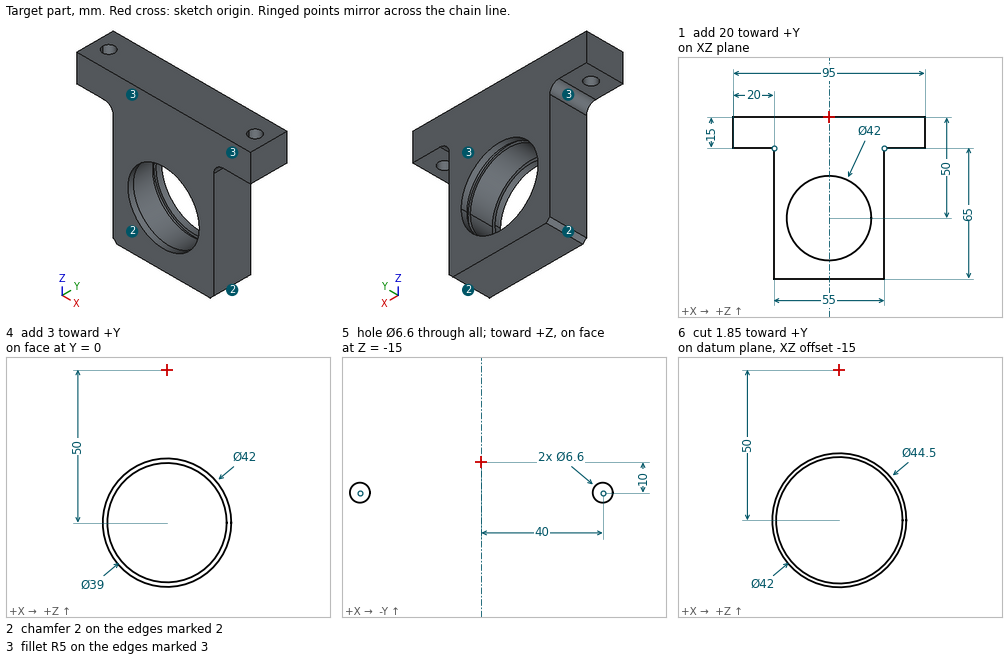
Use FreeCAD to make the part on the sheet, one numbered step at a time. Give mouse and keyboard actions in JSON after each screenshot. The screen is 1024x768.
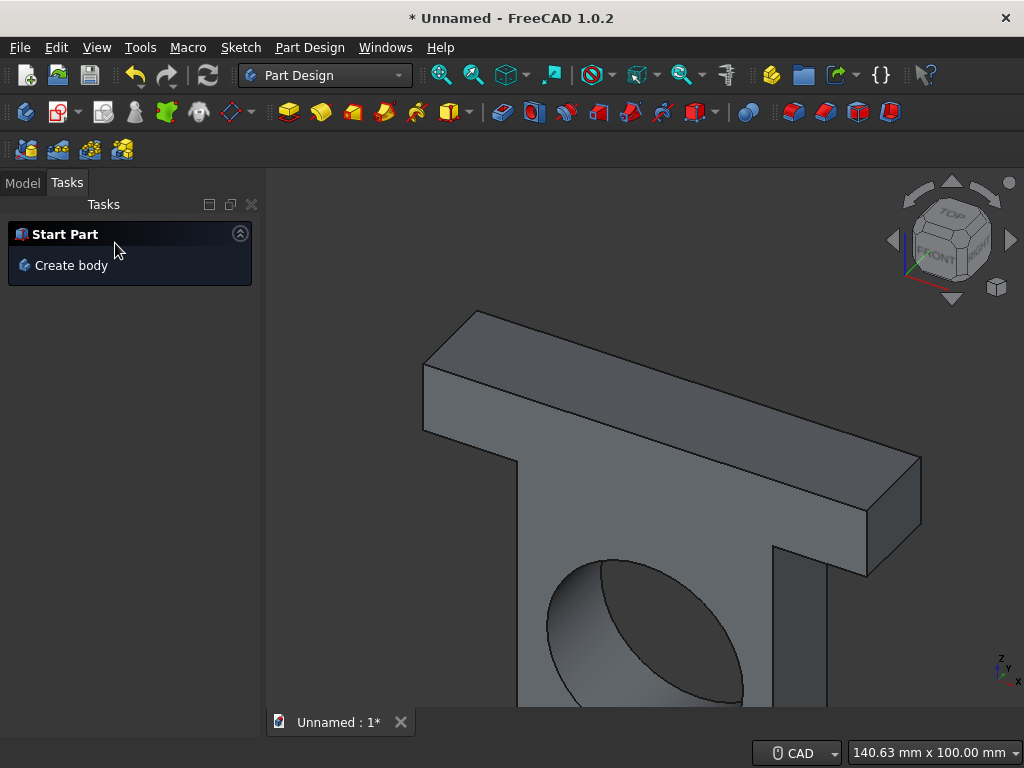
{"action": "left_click", "coordinate": [442, 76]}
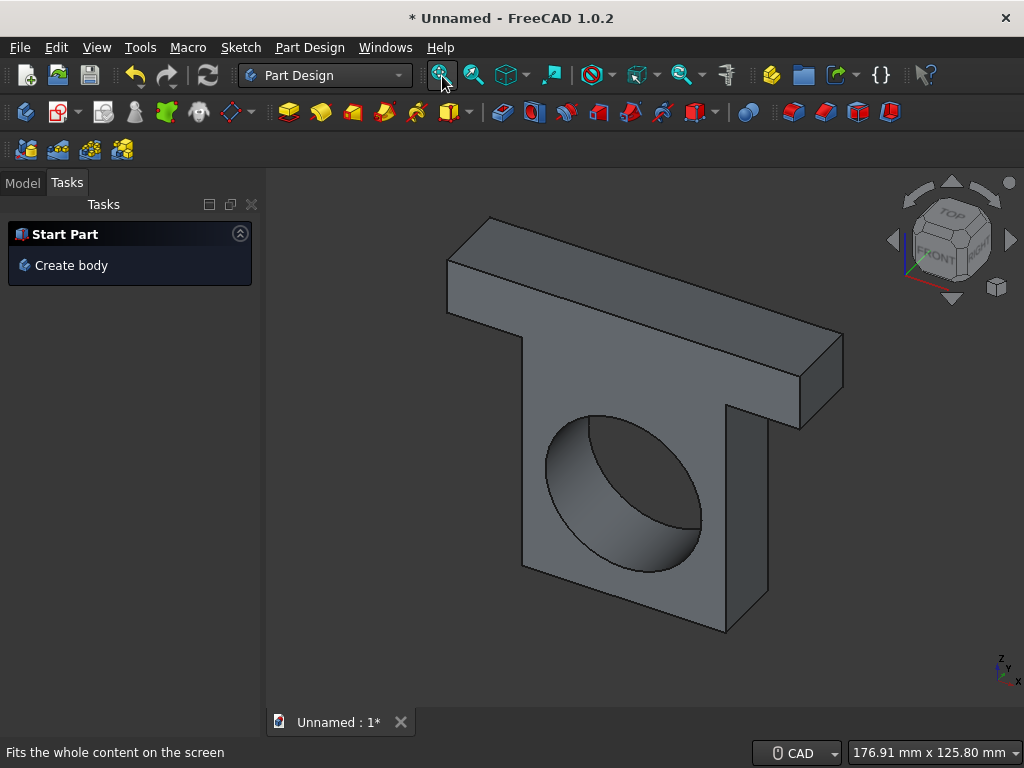
{"action": "key", "text": "0"}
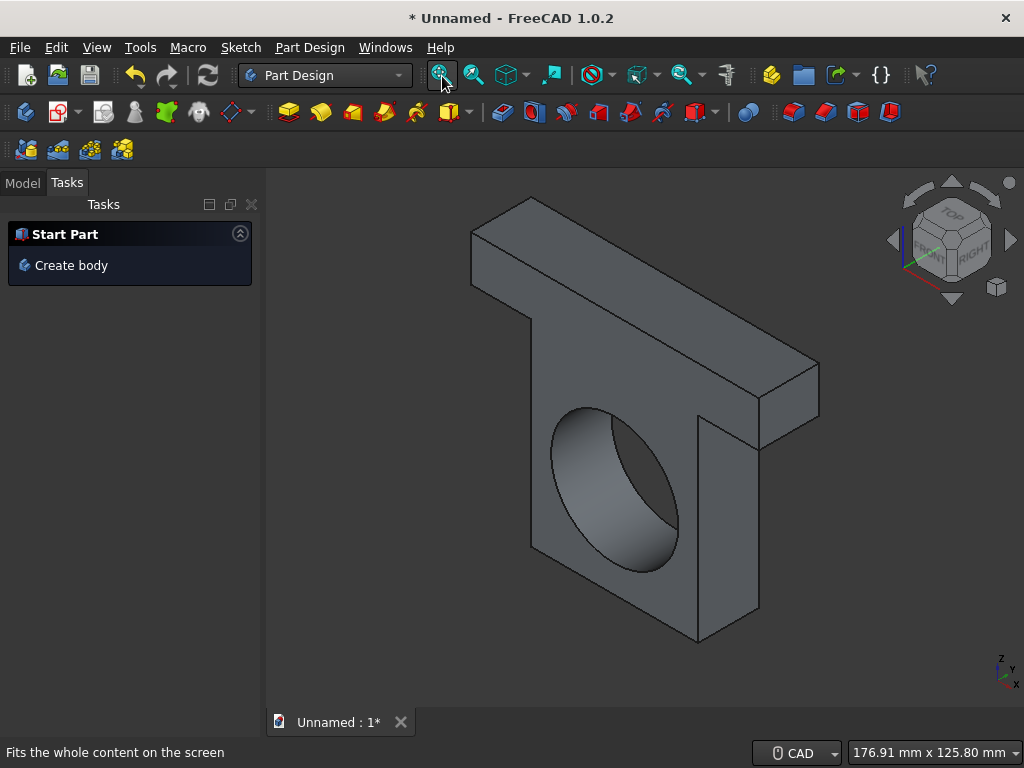
{"action": "key", "text": "2"}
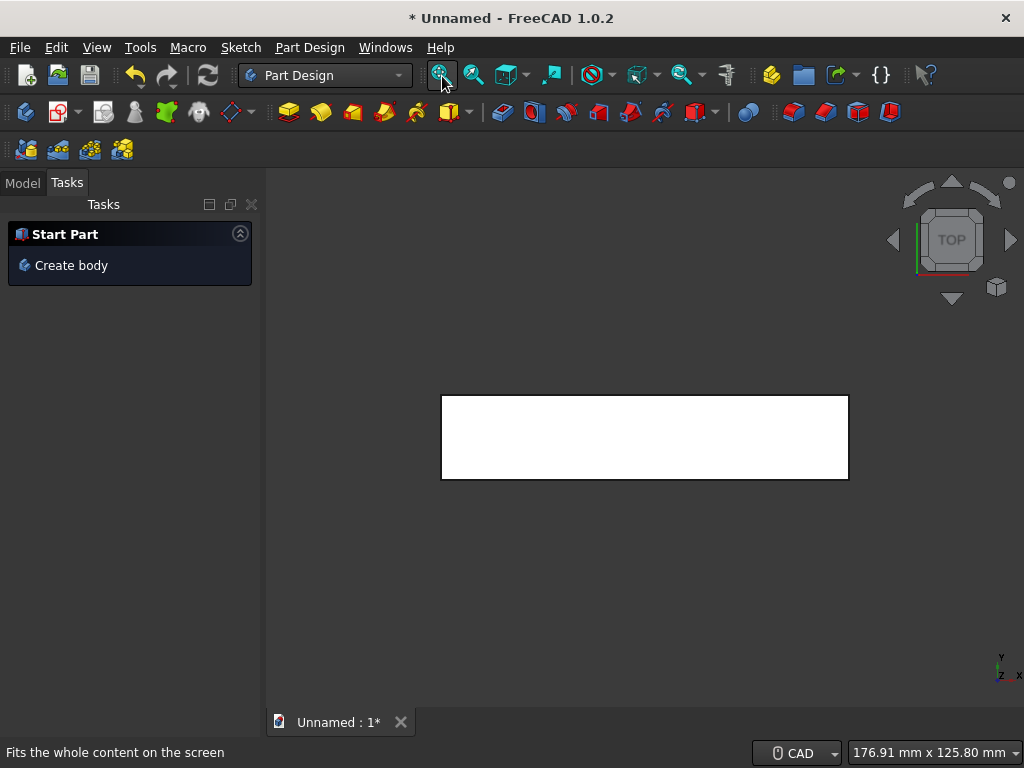
{"action": "key", "text": "1"}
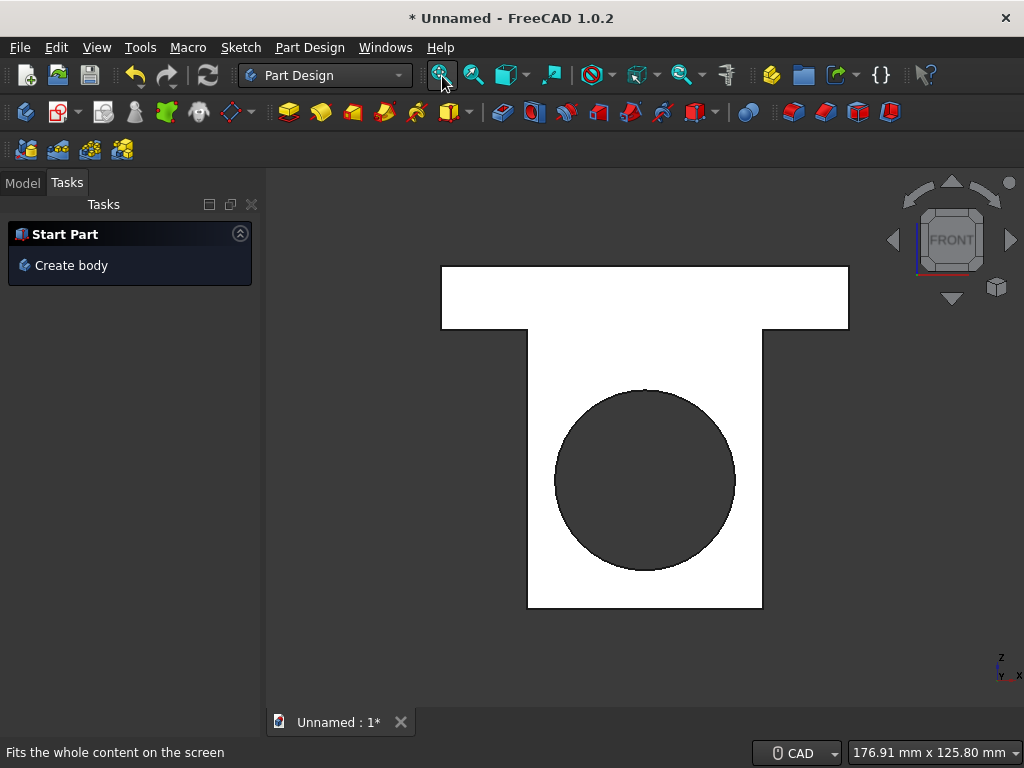
{"action": "key", "text": "3"}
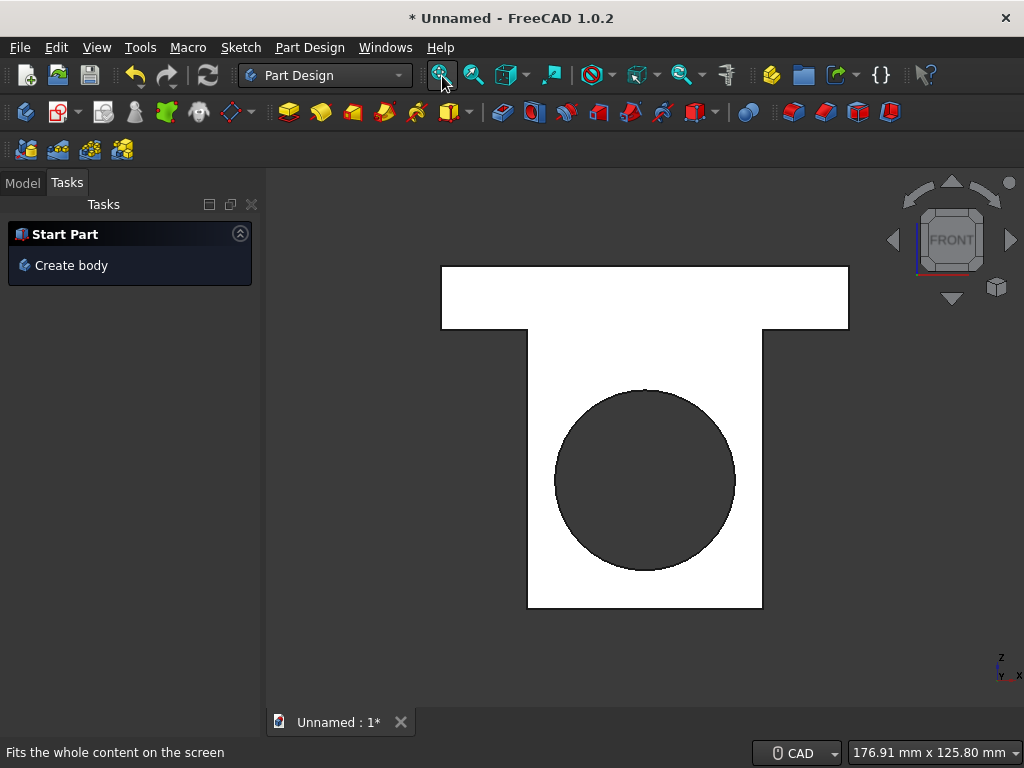
{"action": "left_click", "coordinate": [645, 608]}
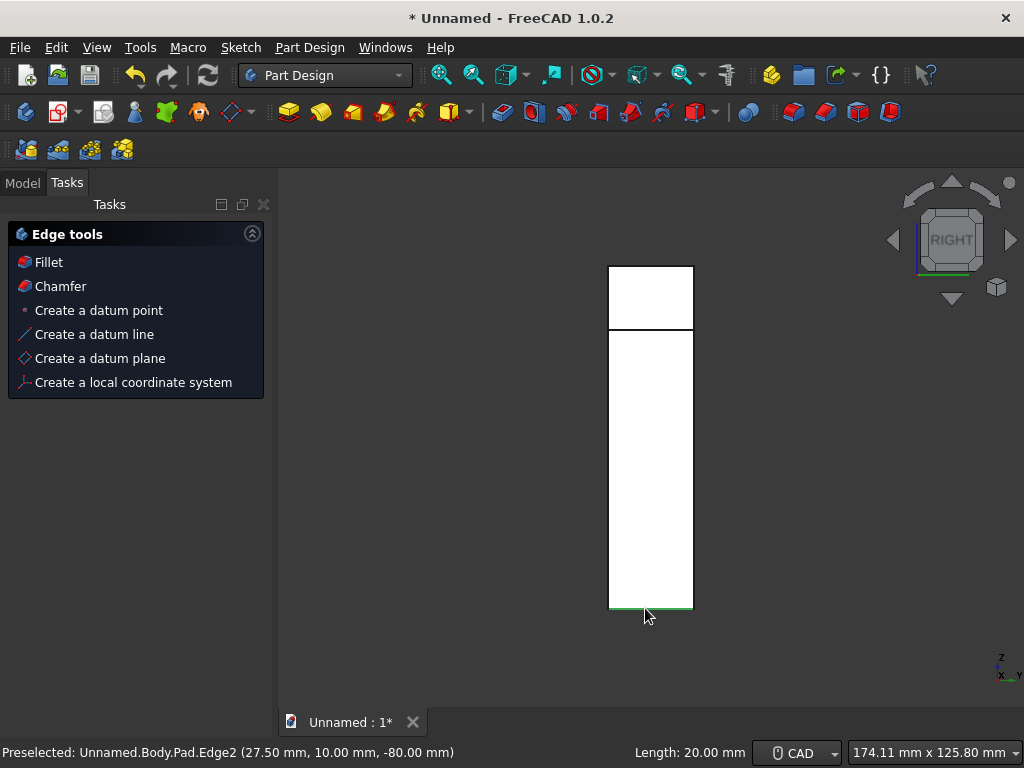
{"action": "key", "text": "5"}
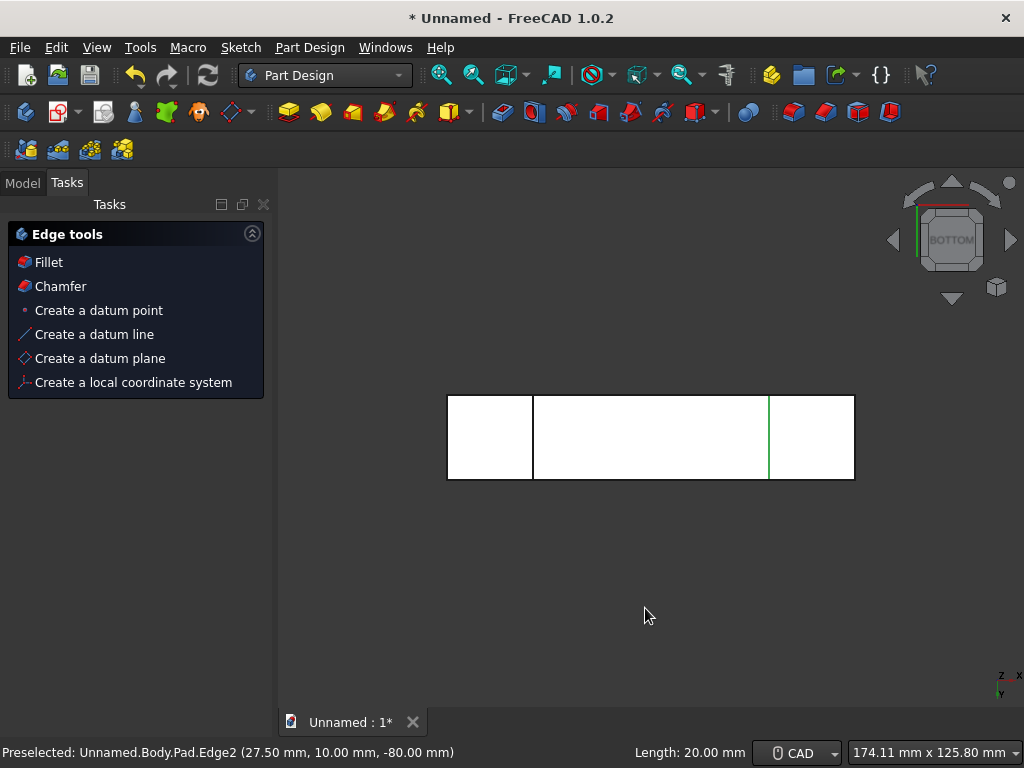
{"action": "left_click", "coordinate": [533, 436], "text": "ctrl"}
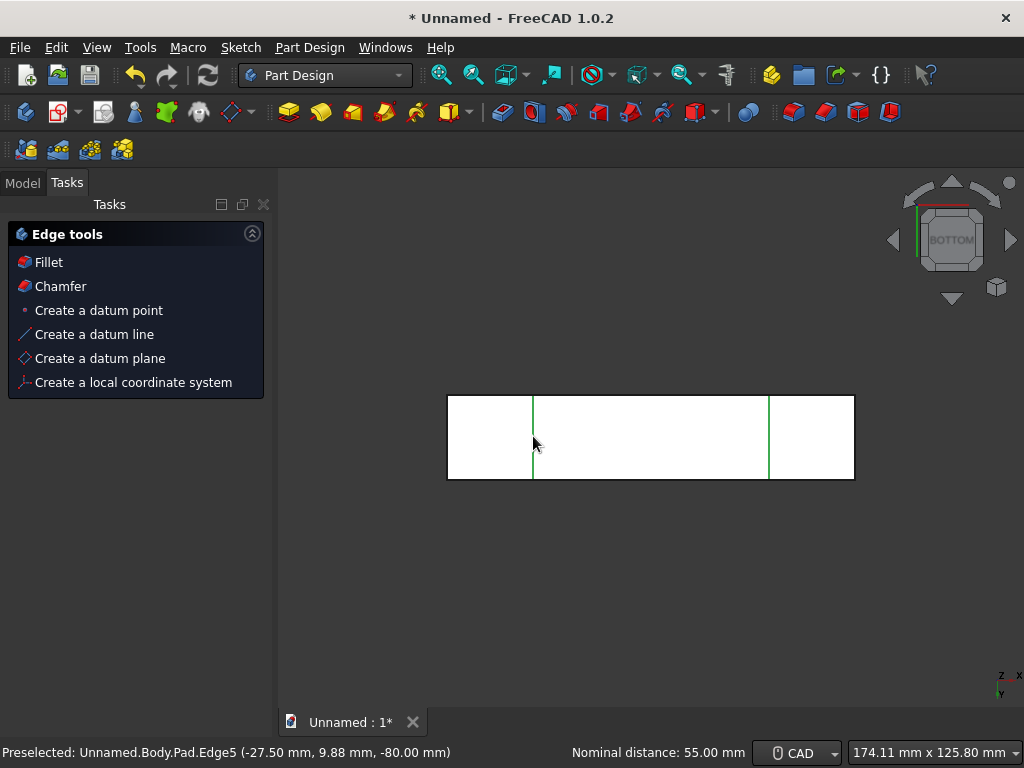
{"action": "left_click", "coordinate": [826, 112]}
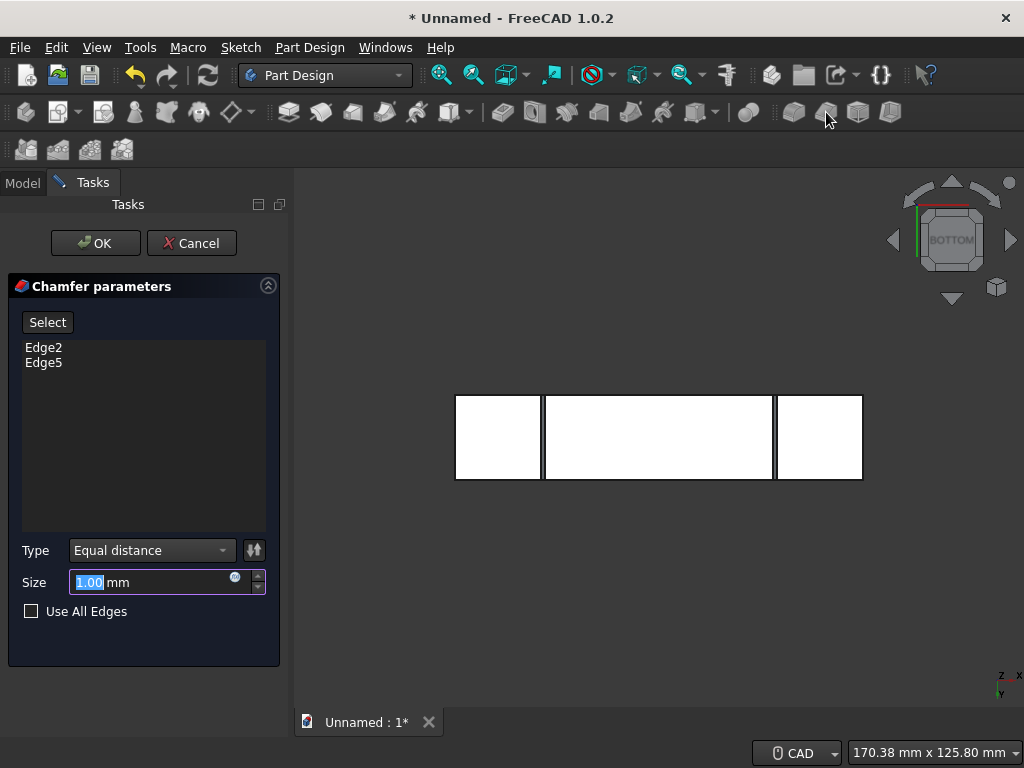
{"action": "type", "text": "2"}
{"action": "key", "text": "Tab"}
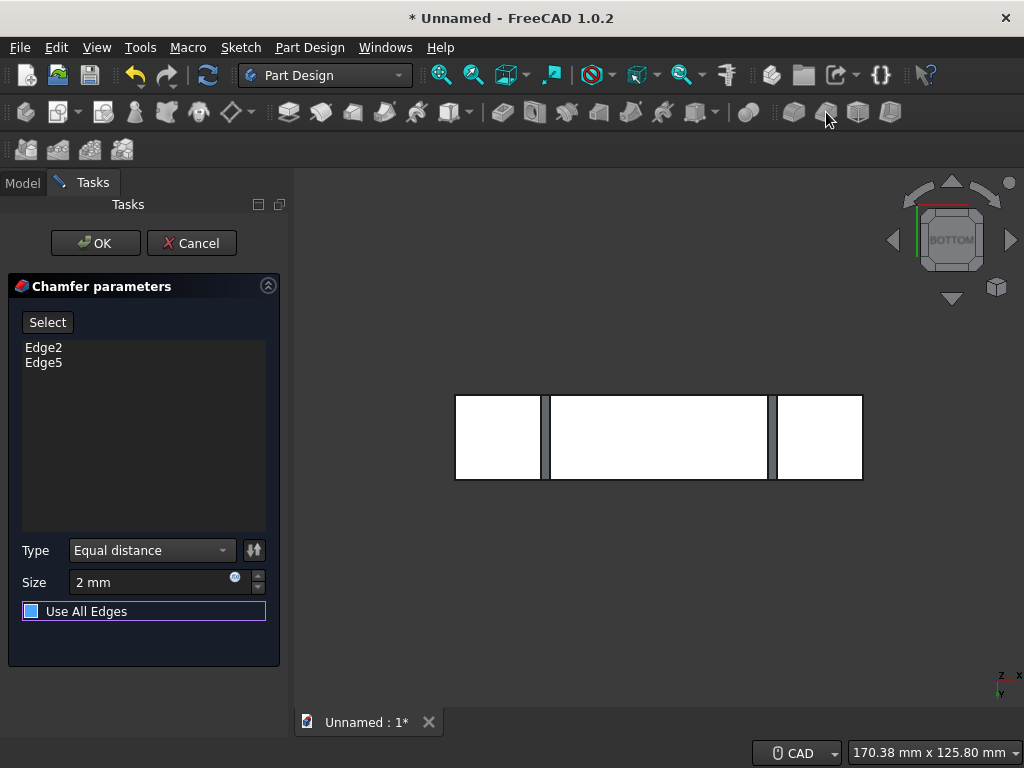
{"action": "left_click", "coordinate": [96, 243]}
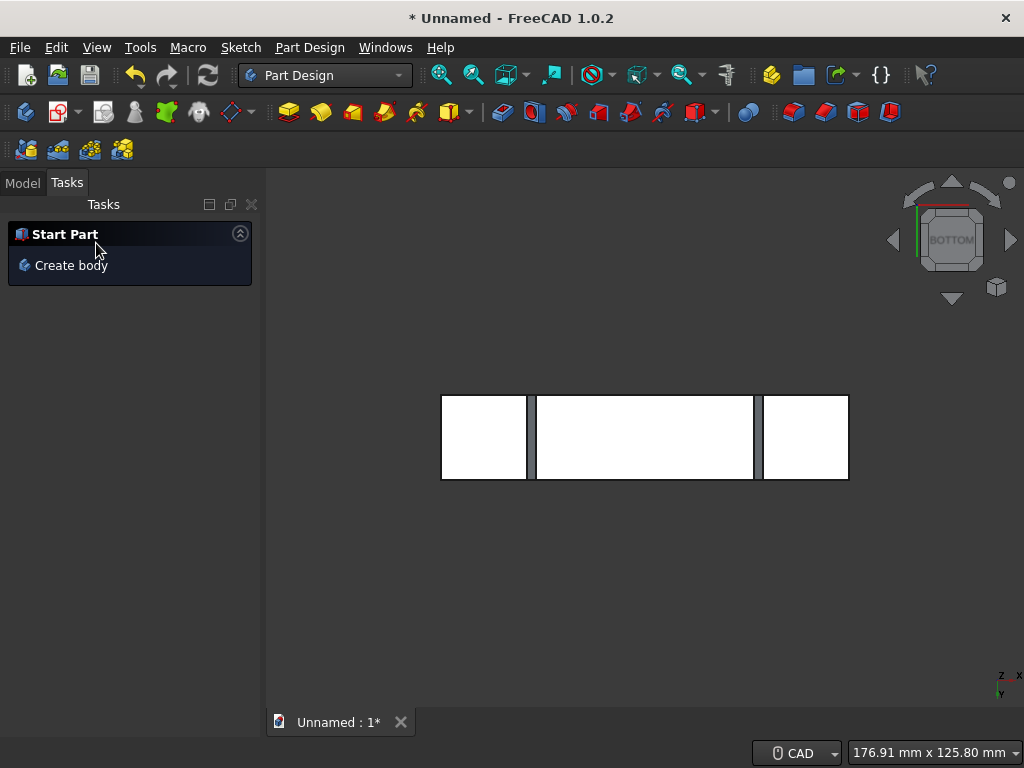
{"action": "key", "text": "0"}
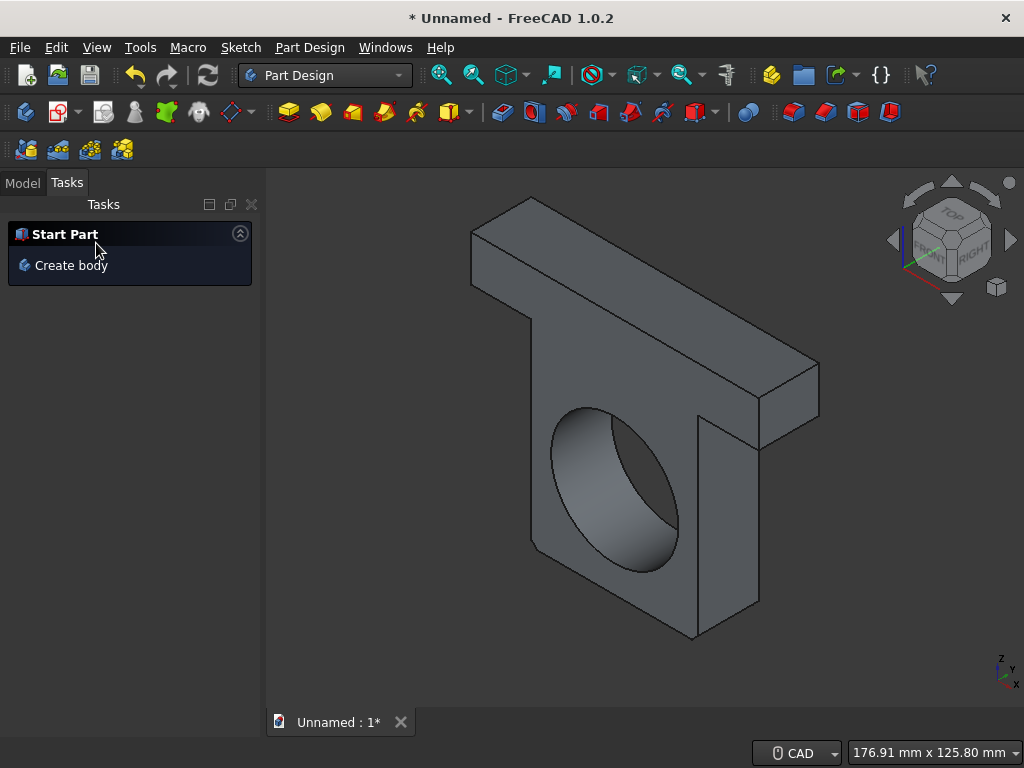
{"action": "key", "text": "2"}